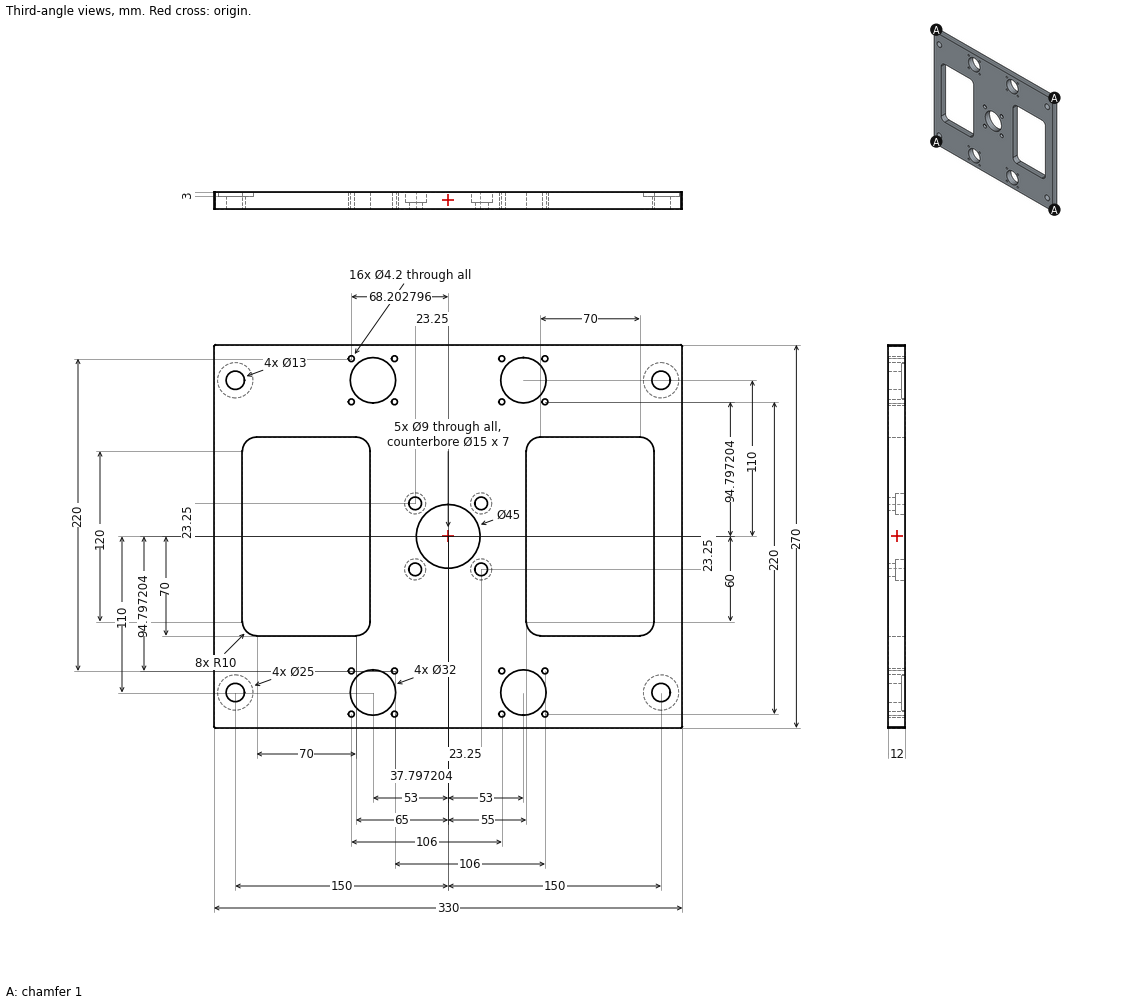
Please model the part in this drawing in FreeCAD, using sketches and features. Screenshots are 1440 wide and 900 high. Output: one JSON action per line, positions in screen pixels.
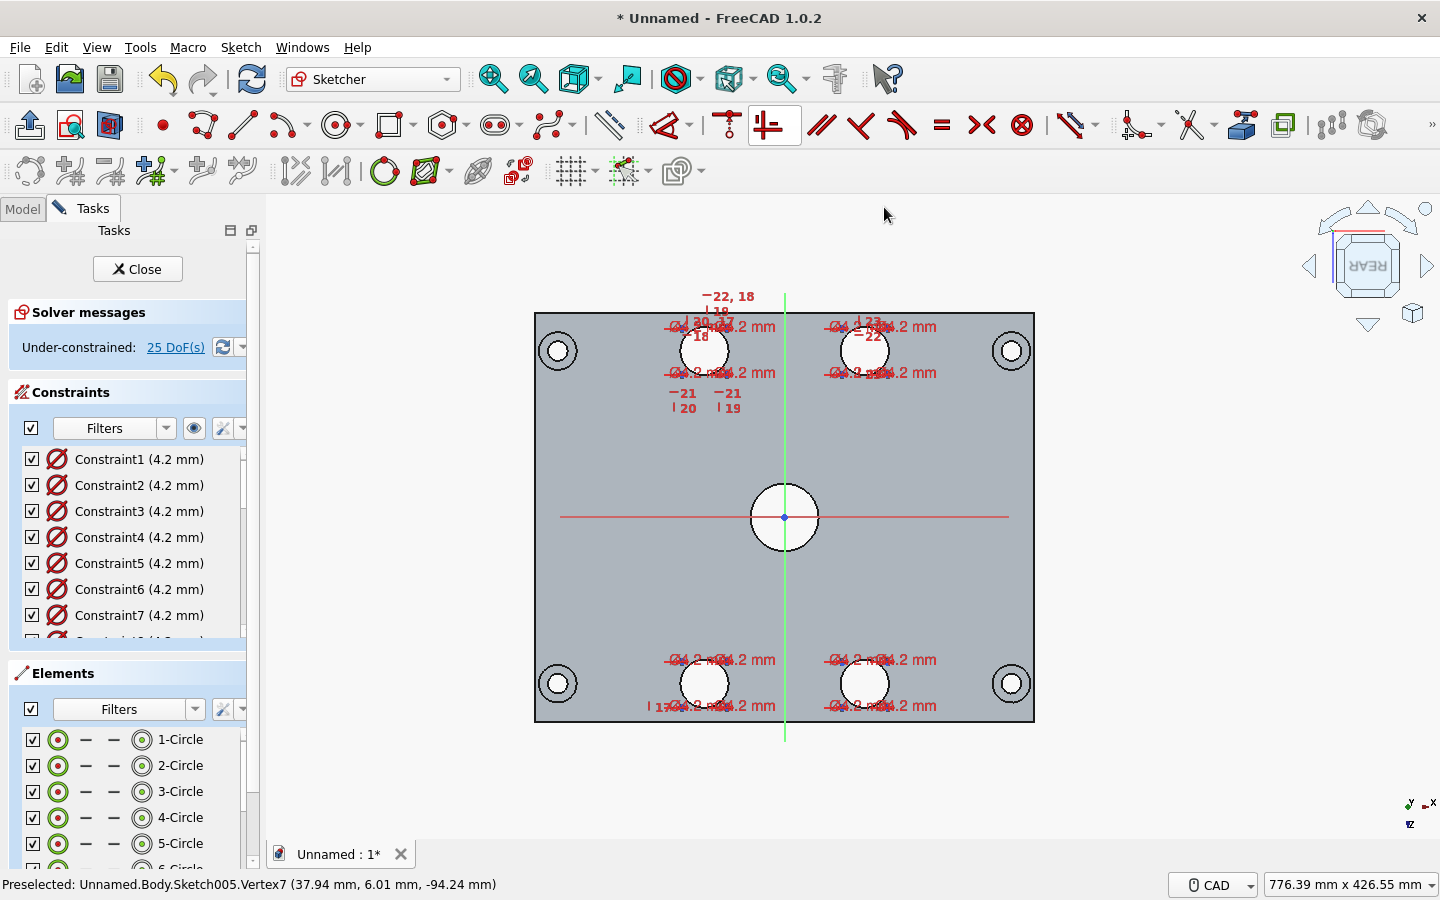
{"action": "left_click", "coordinate": [727, 375]}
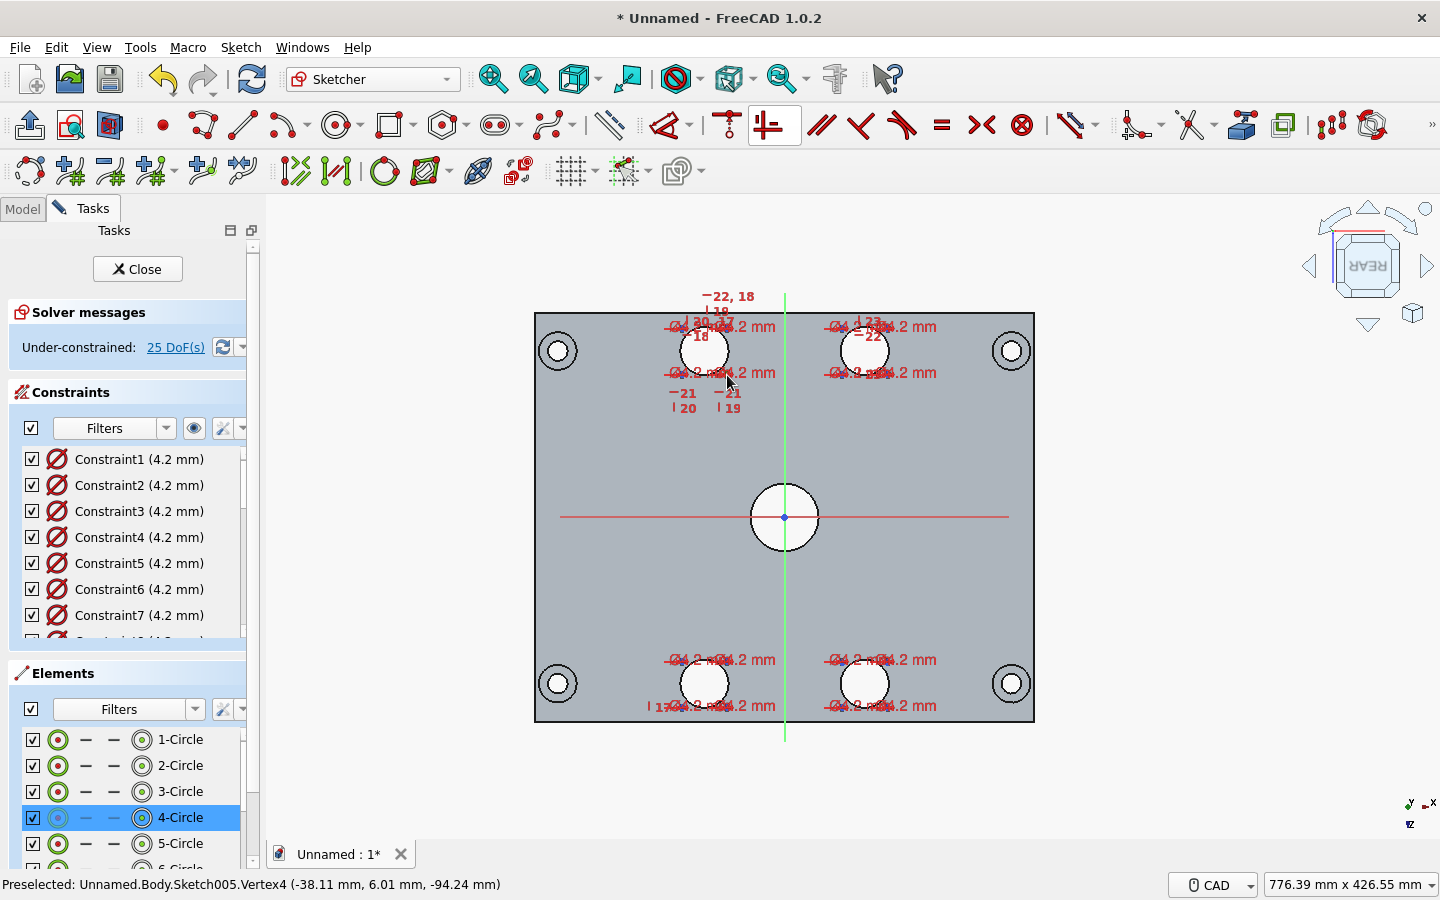
{"action": "left_click", "coordinate": [842, 375]}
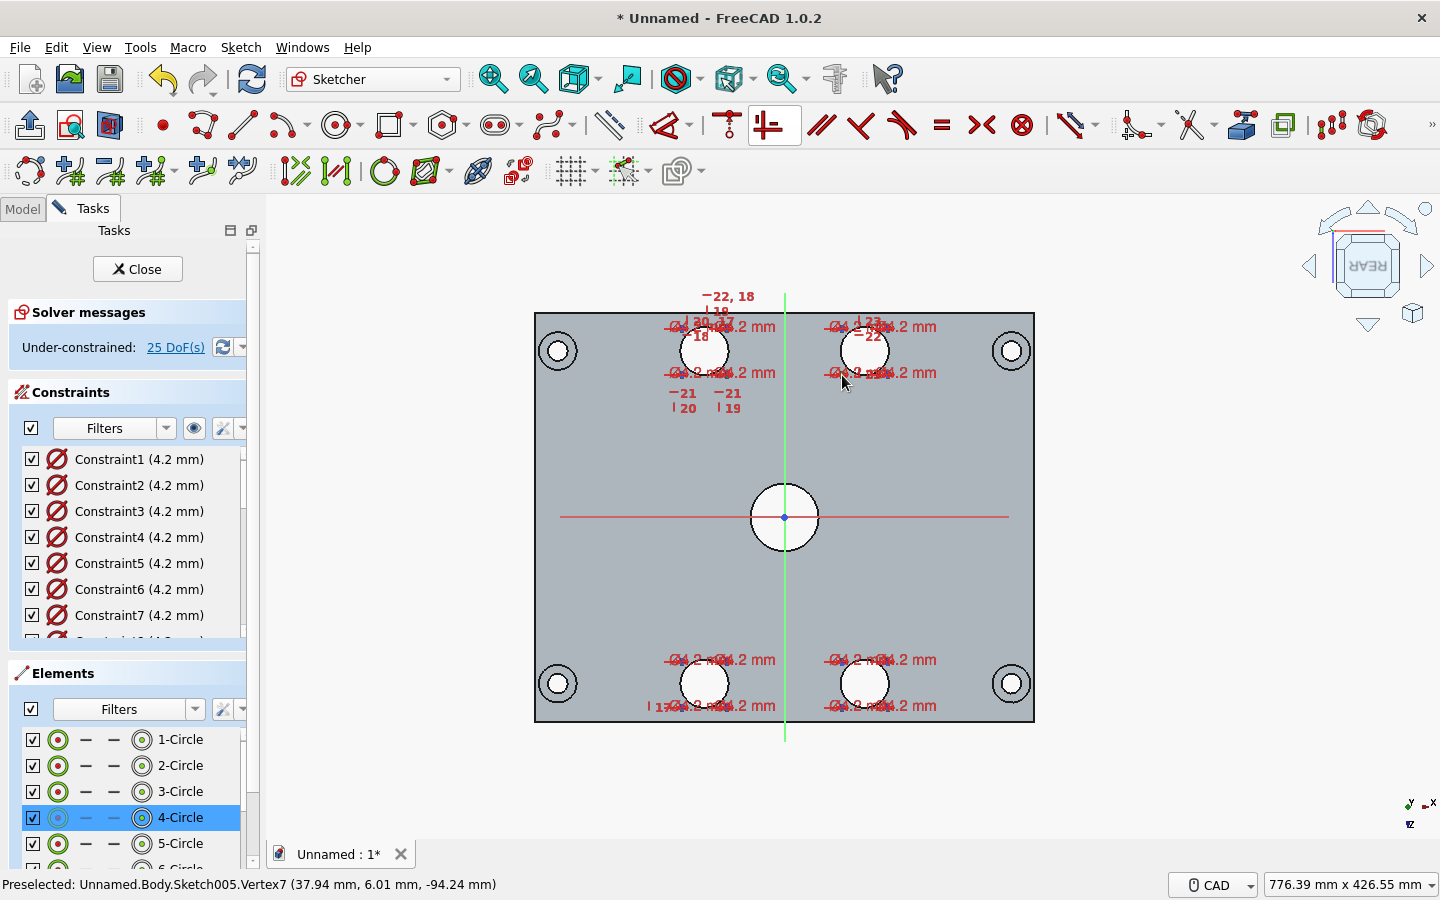
{"action": "left_click", "coordinate": [796, 126]}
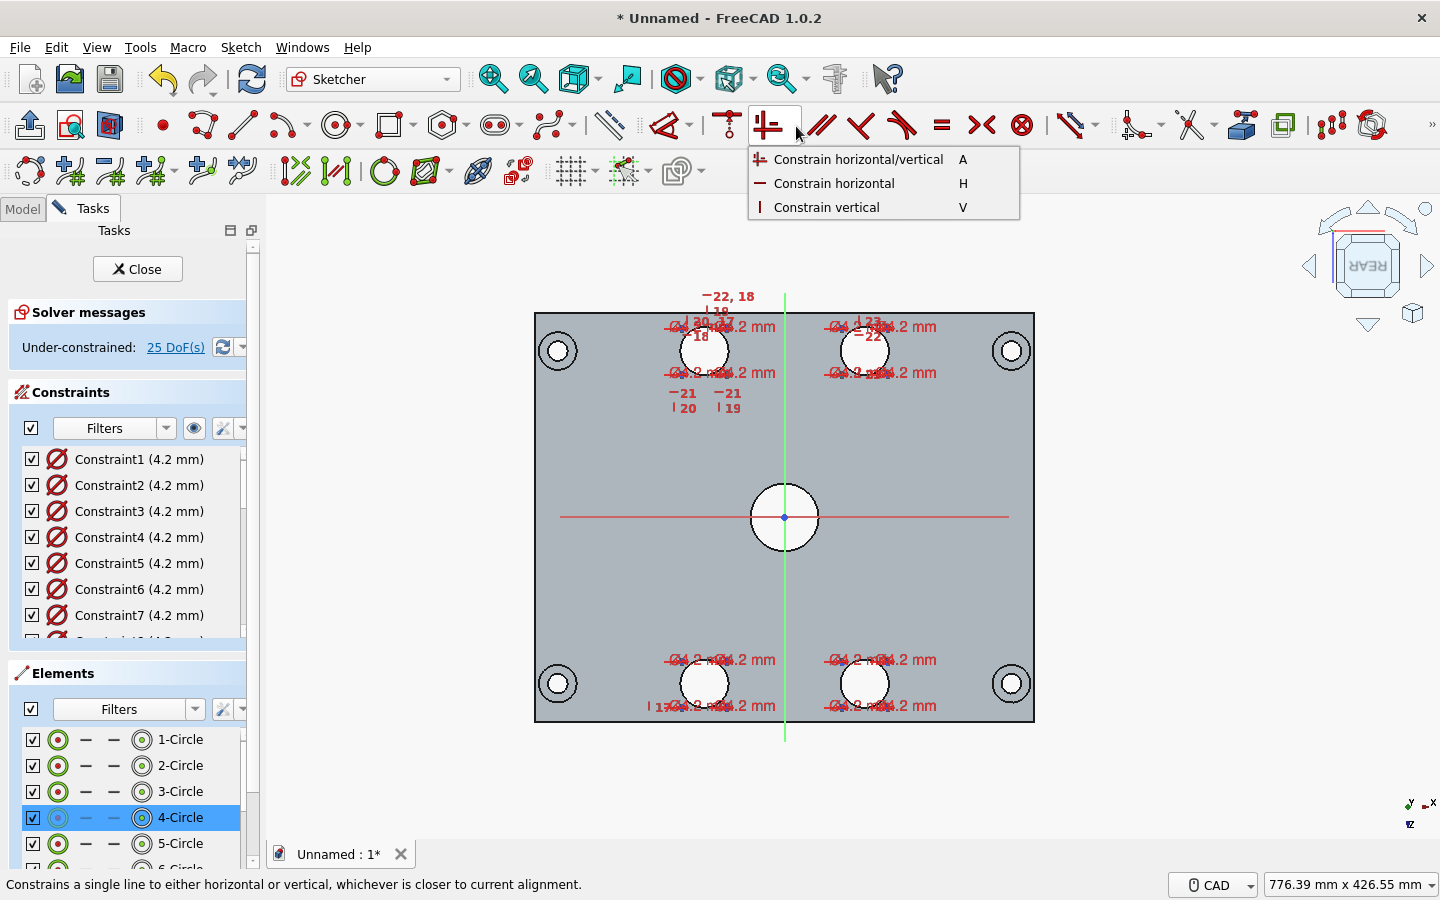
{"action": "left_click", "coordinate": [884, 183]}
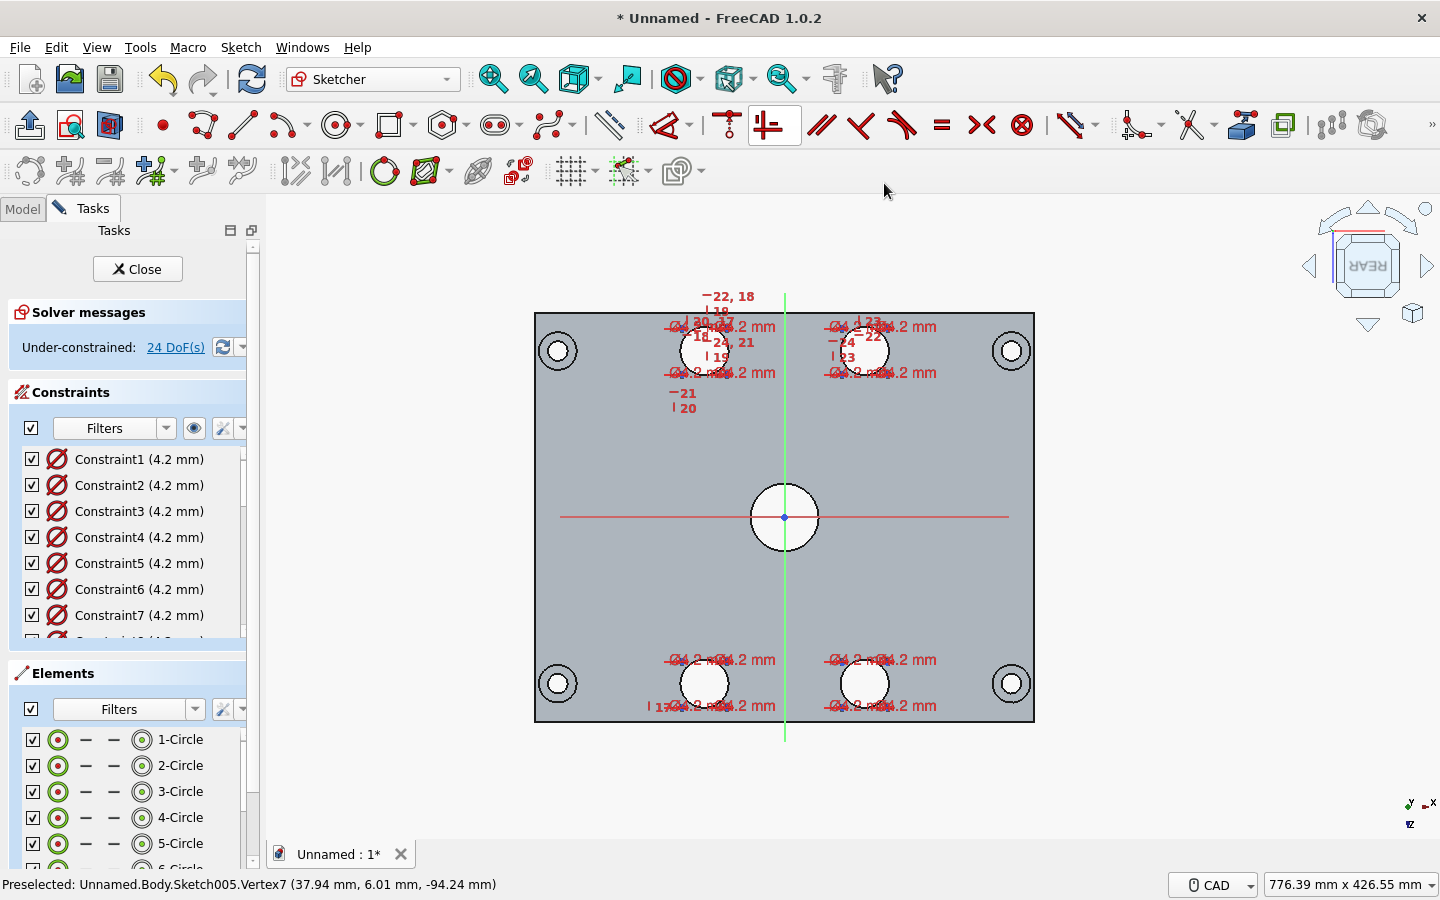
{"action": "left_click", "coordinate": [842, 375]}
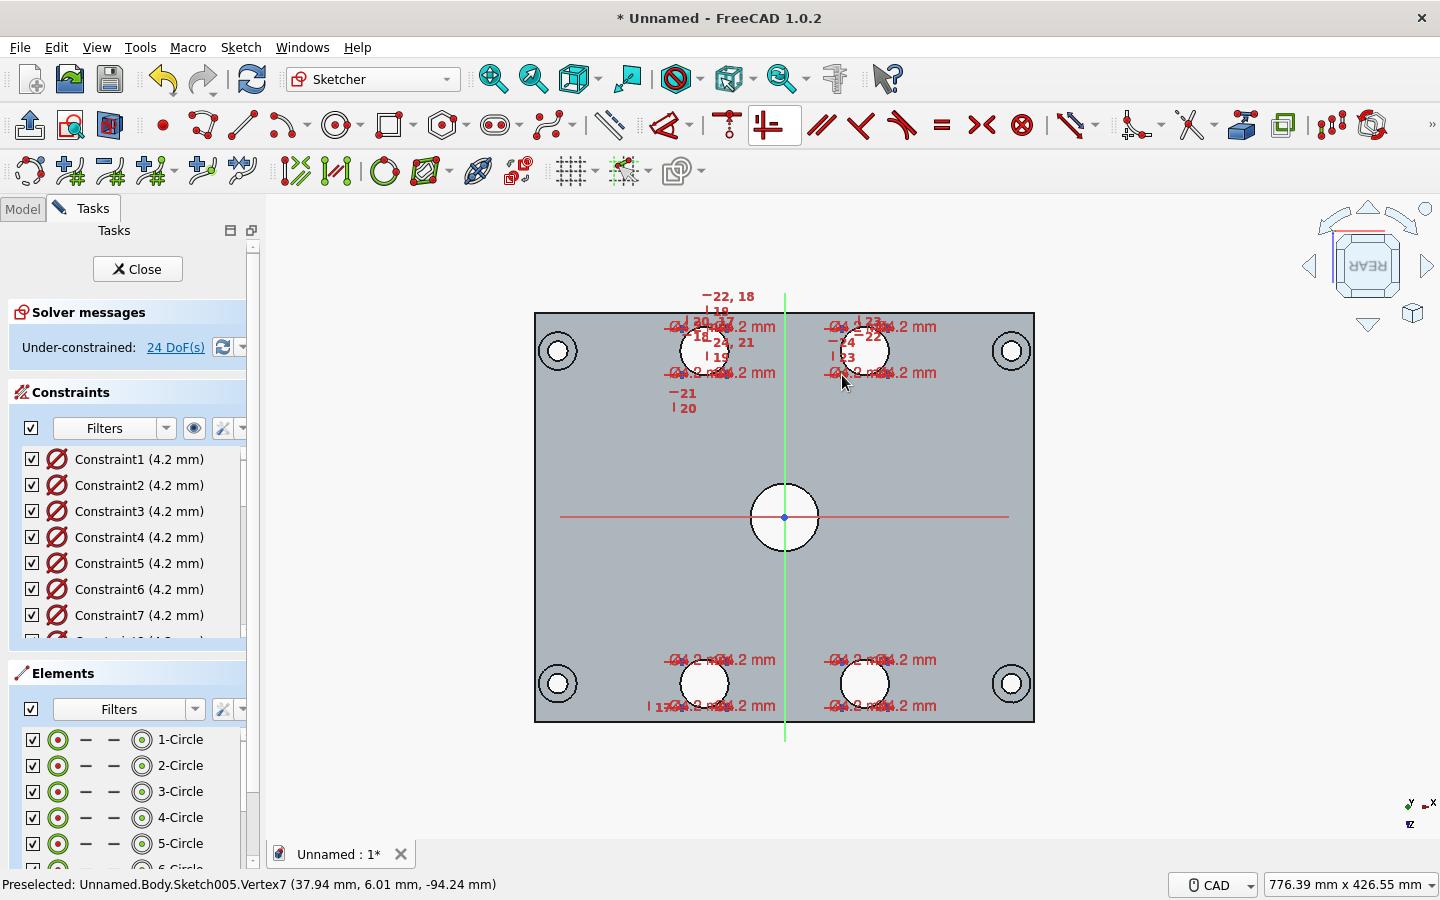
{"action": "left_click", "coordinate": [888, 375]}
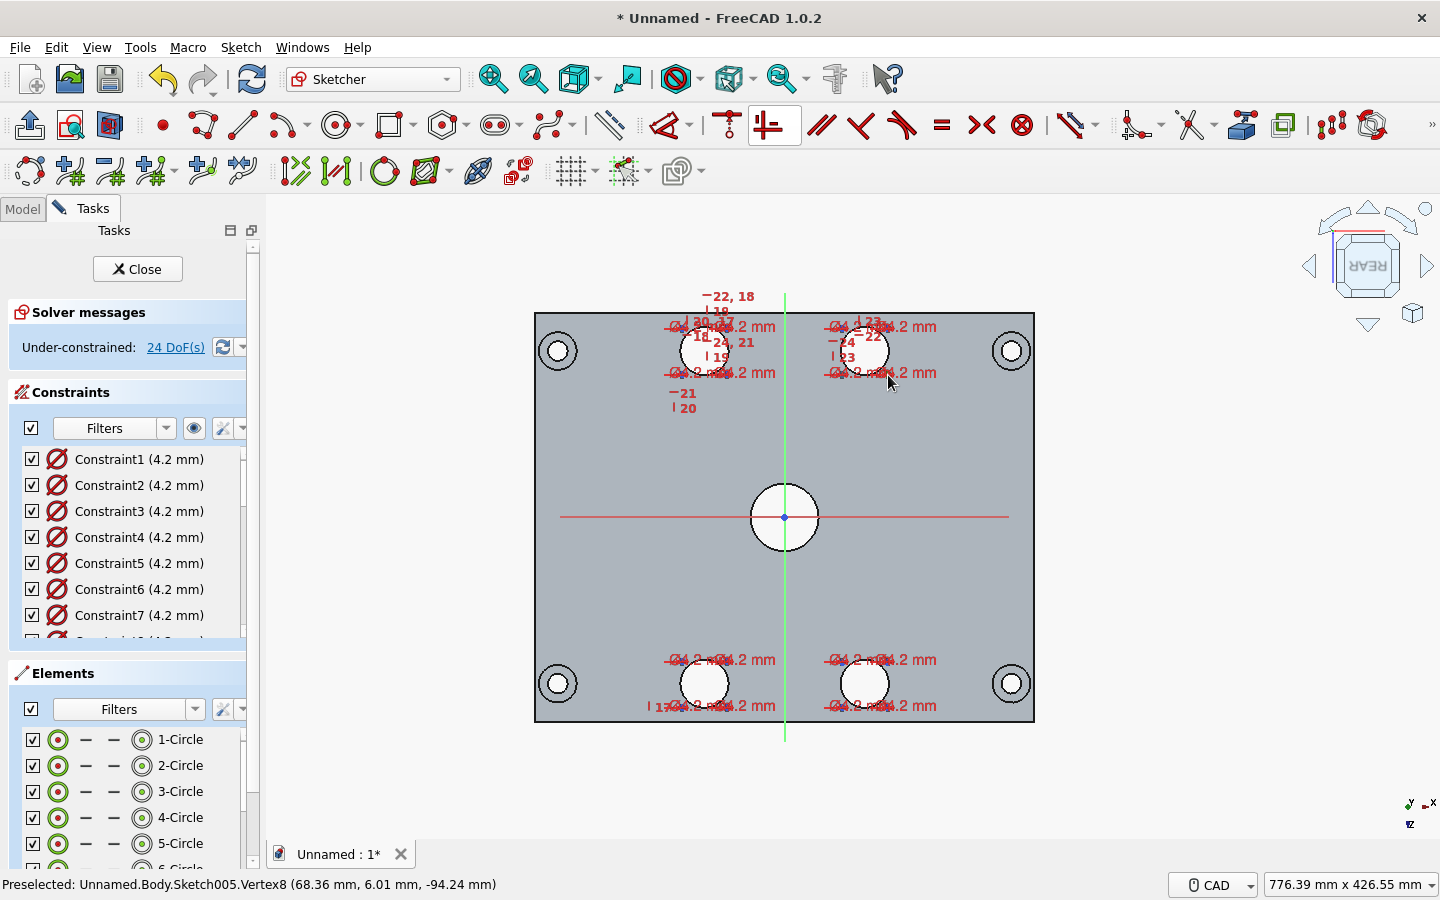
{"action": "key", "text": "h"}